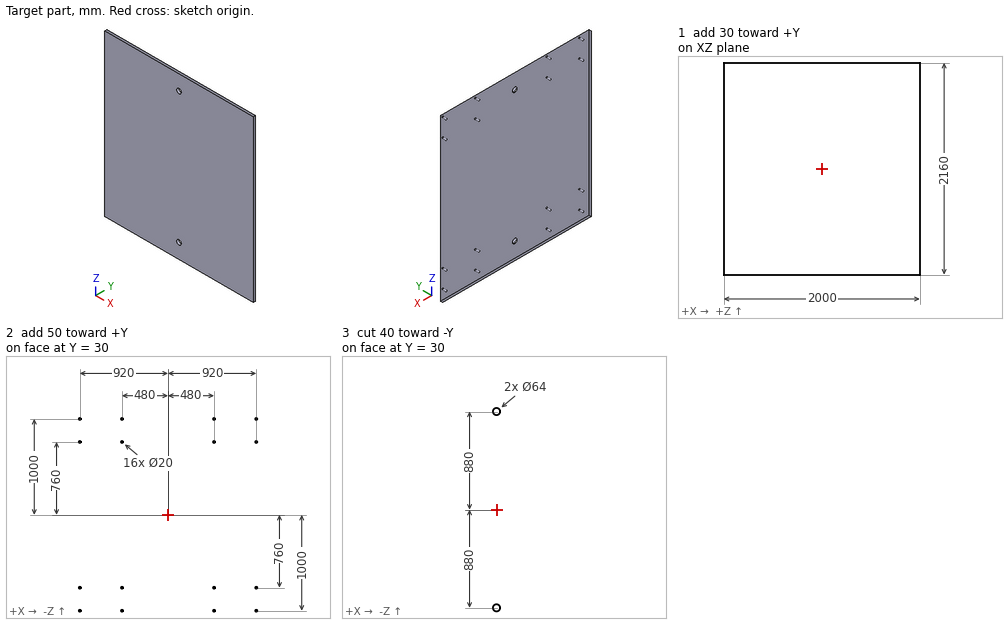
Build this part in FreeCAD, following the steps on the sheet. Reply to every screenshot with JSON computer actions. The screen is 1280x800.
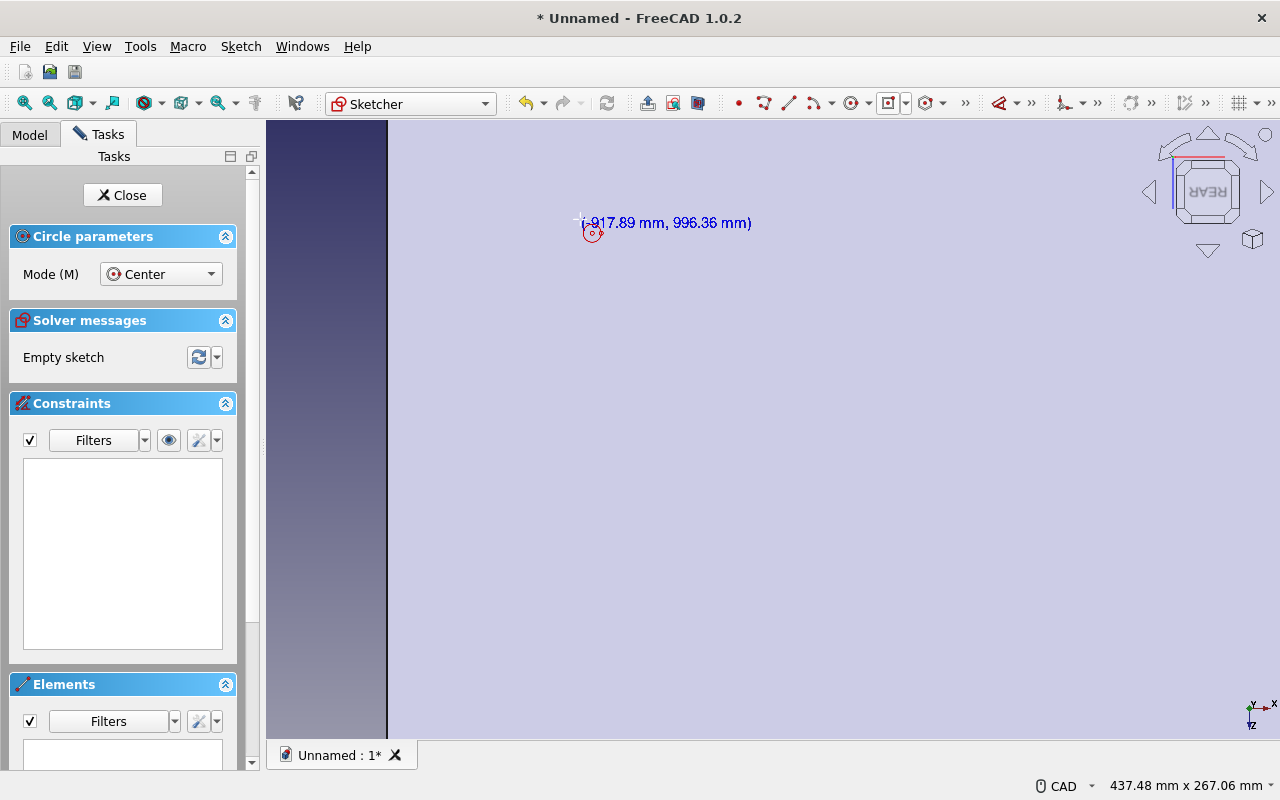
{"action": "scroll", "coordinate": [505, 219], "scroll_direction": "down", "scroll_amount": 12}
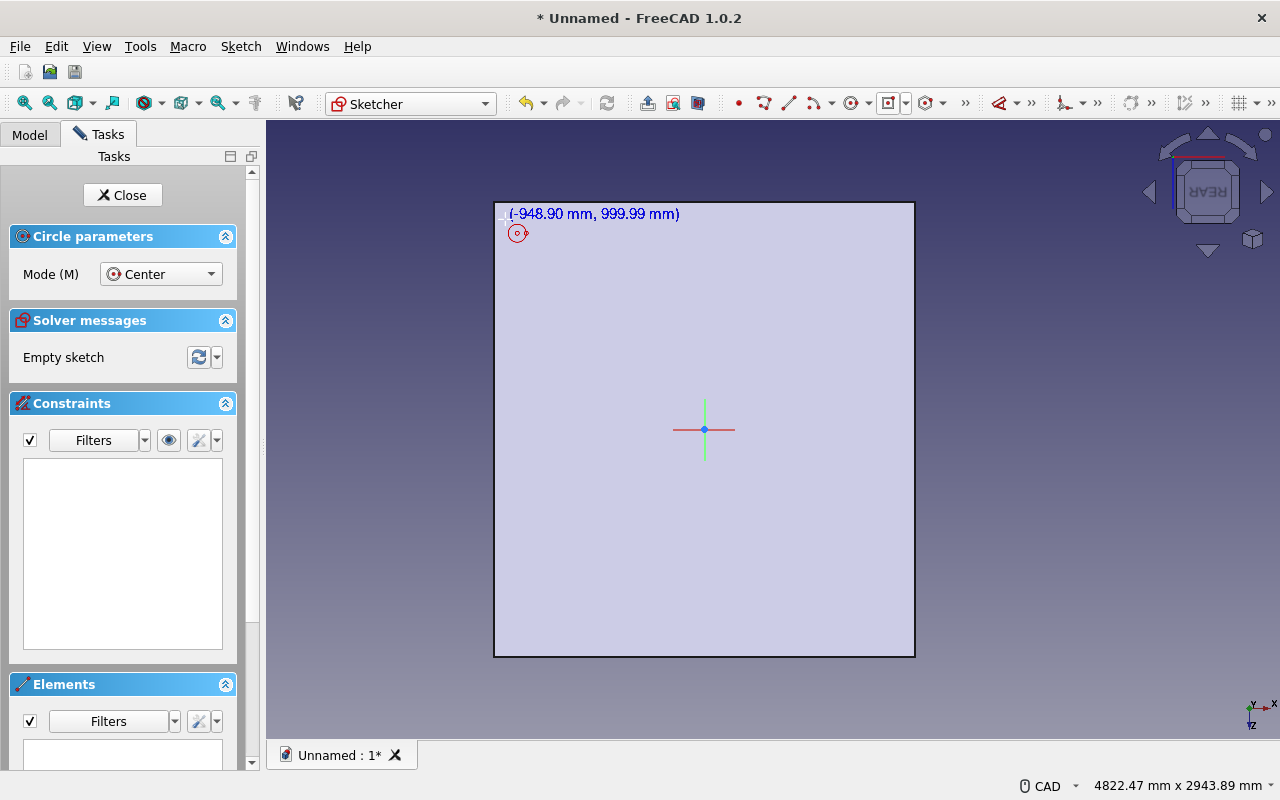
{"action": "left_click", "coordinate": [511, 219]}
{"action": "mouse_move", "coordinate": [513, 218]}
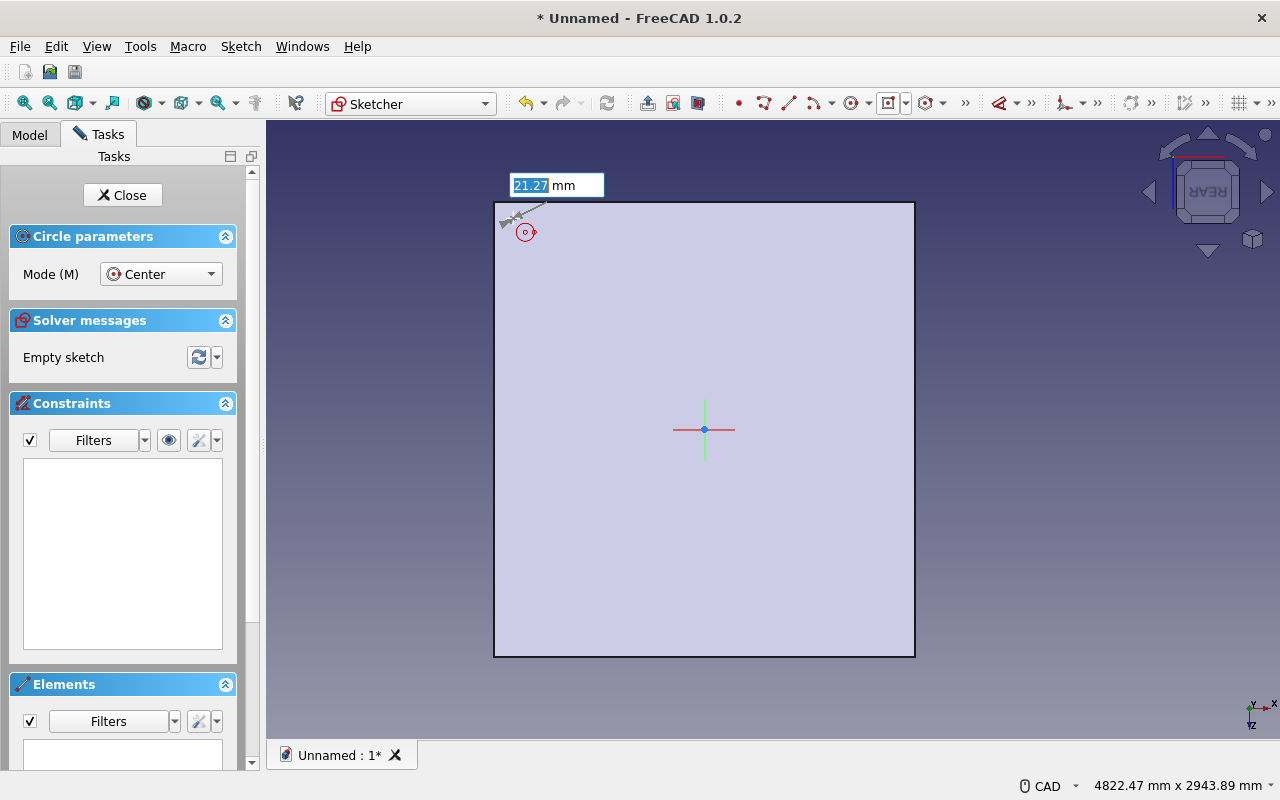
{"action": "type", "text": "20"}
{"action": "key", "text": "Return"}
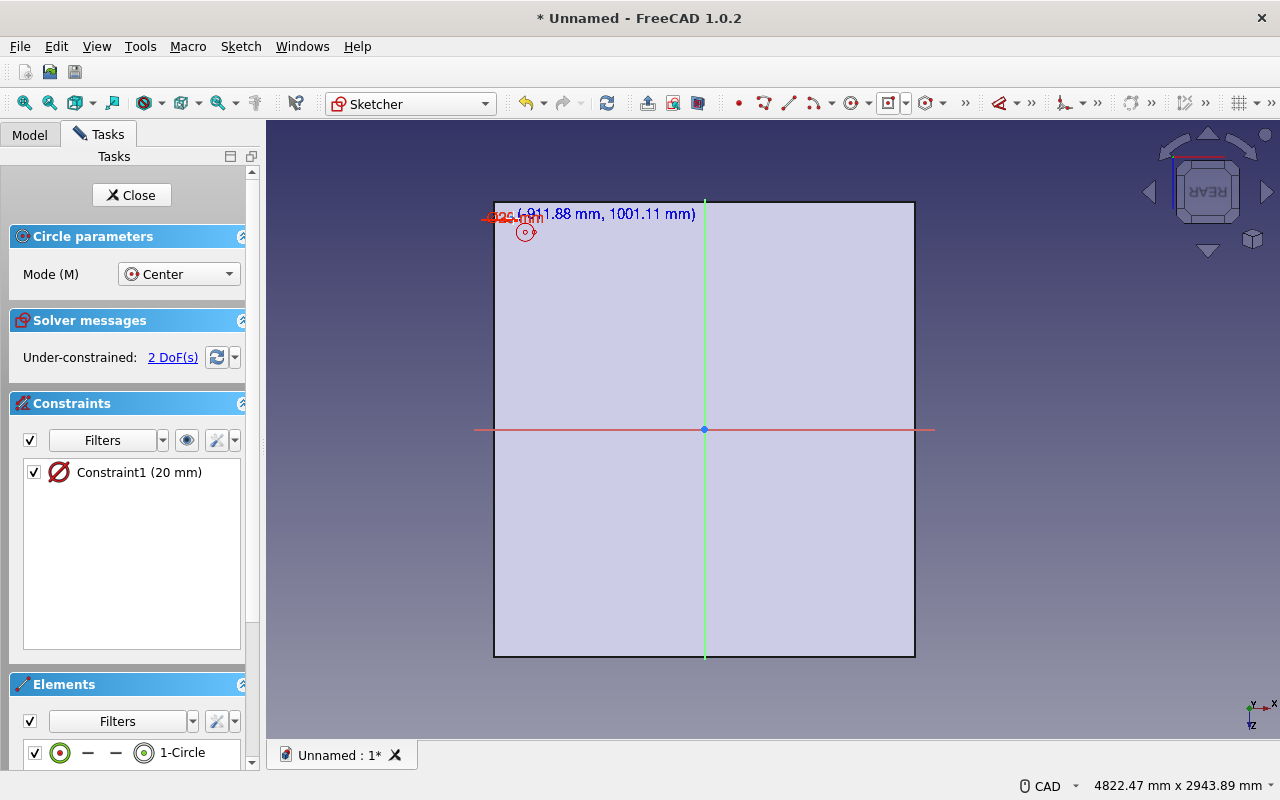
{"action": "scroll", "coordinate": [511, 270], "scroll_direction": "up", "scroll_amount": 12}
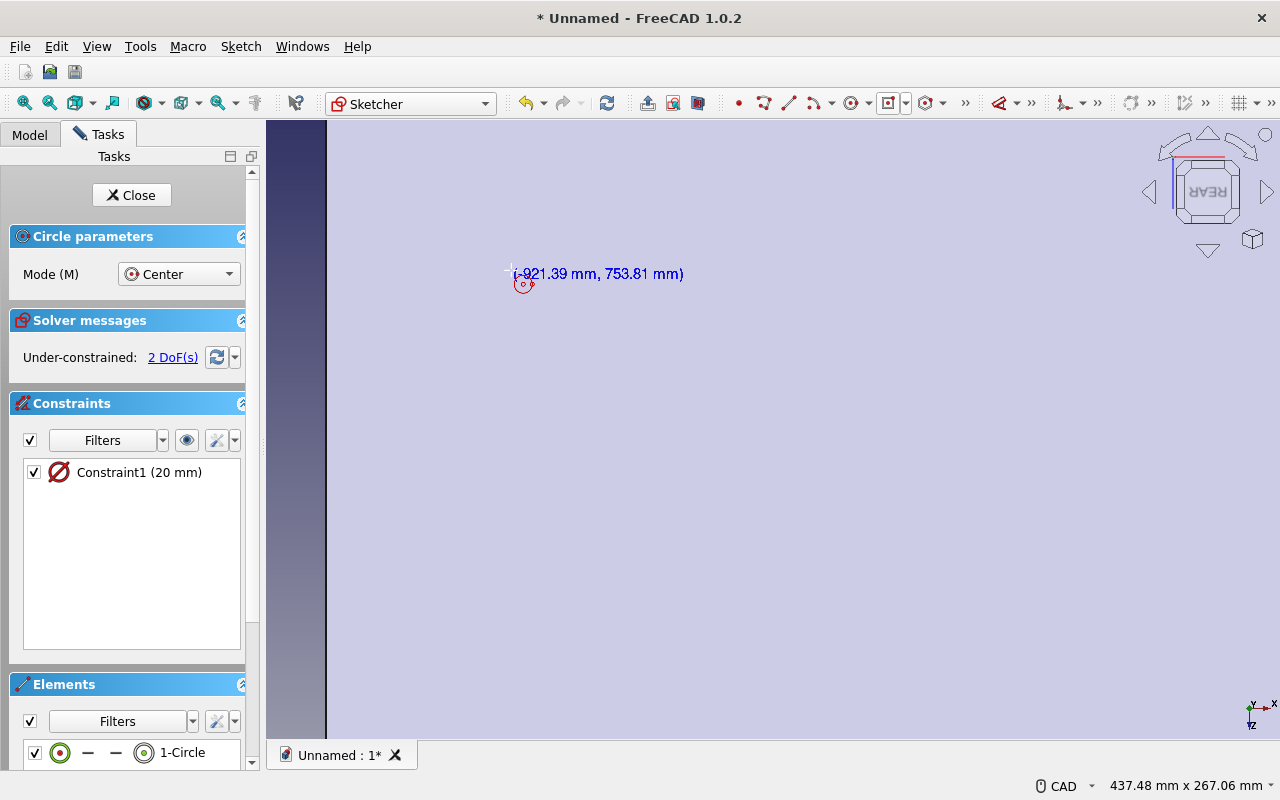
{"action": "scroll", "coordinate": [511, 270], "scroll_direction": "down", "scroll_amount": 12}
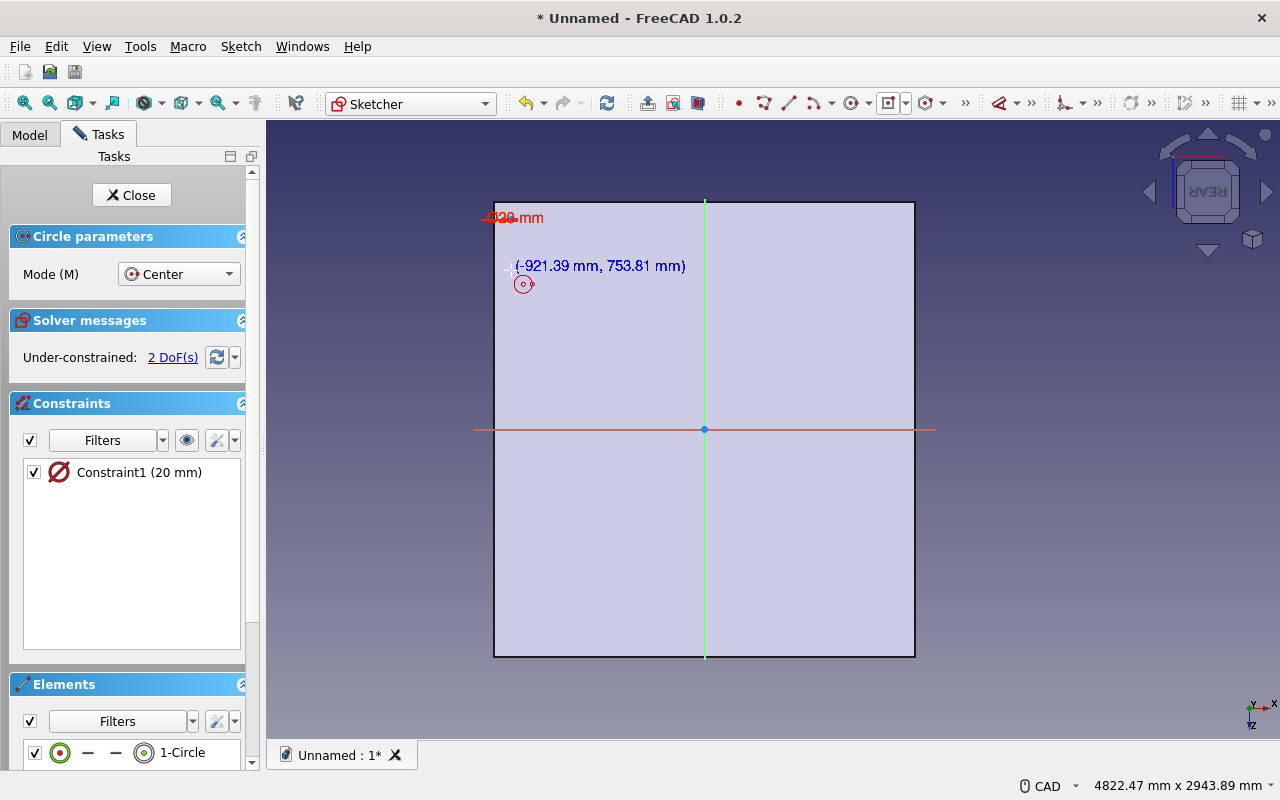
{"action": "left_click", "coordinate": [511, 270]}
{"action": "mouse_move", "coordinate": [513, 268]}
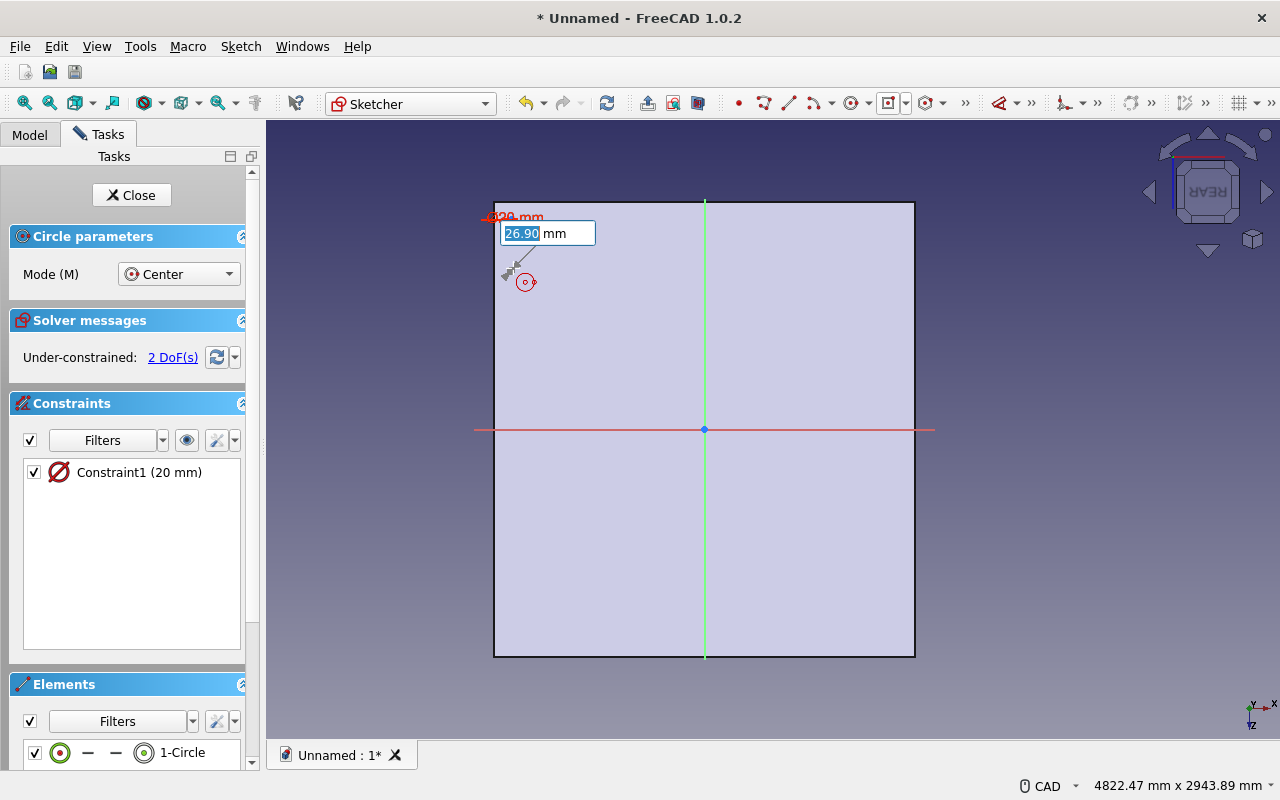
{"action": "type", "text": "20"}
{"action": "key", "text": "Return"}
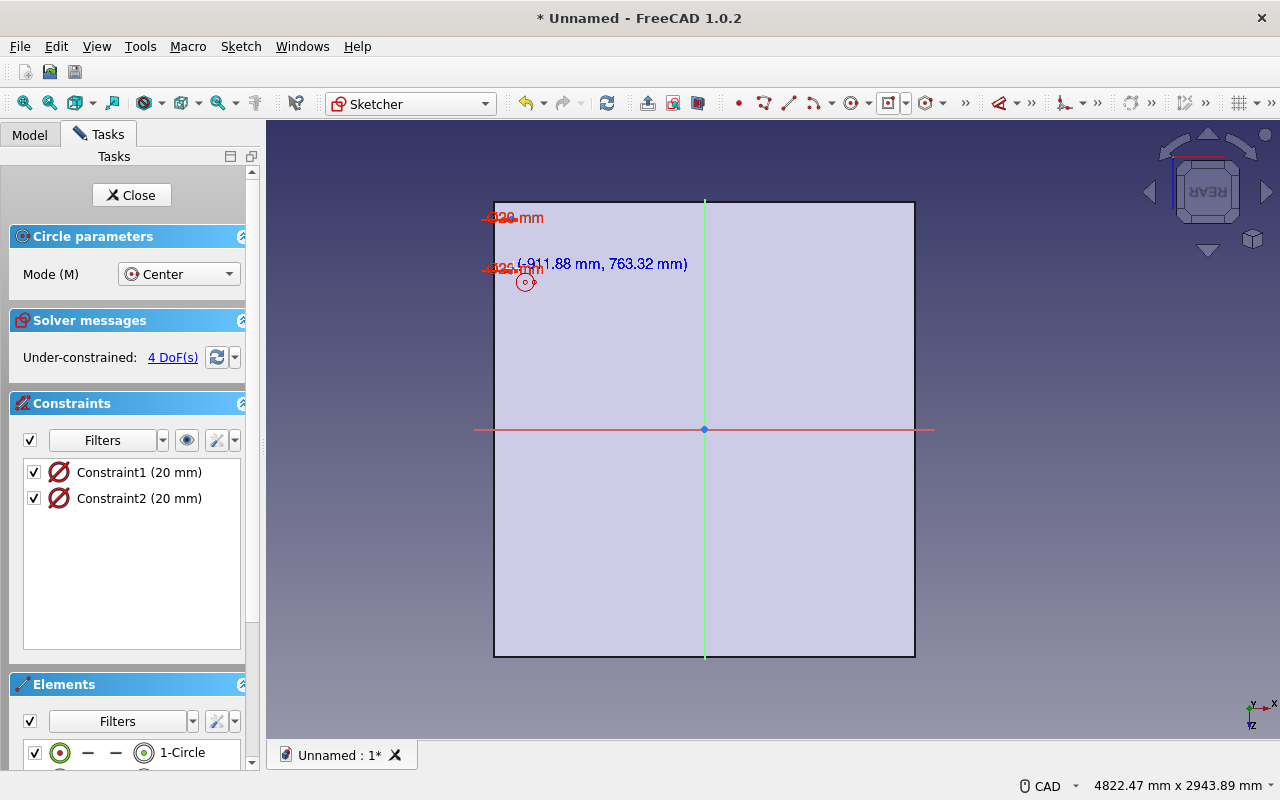
{"action": "scroll", "coordinate": [604, 219], "scroll_direction": "up", "scroll_amount": 12}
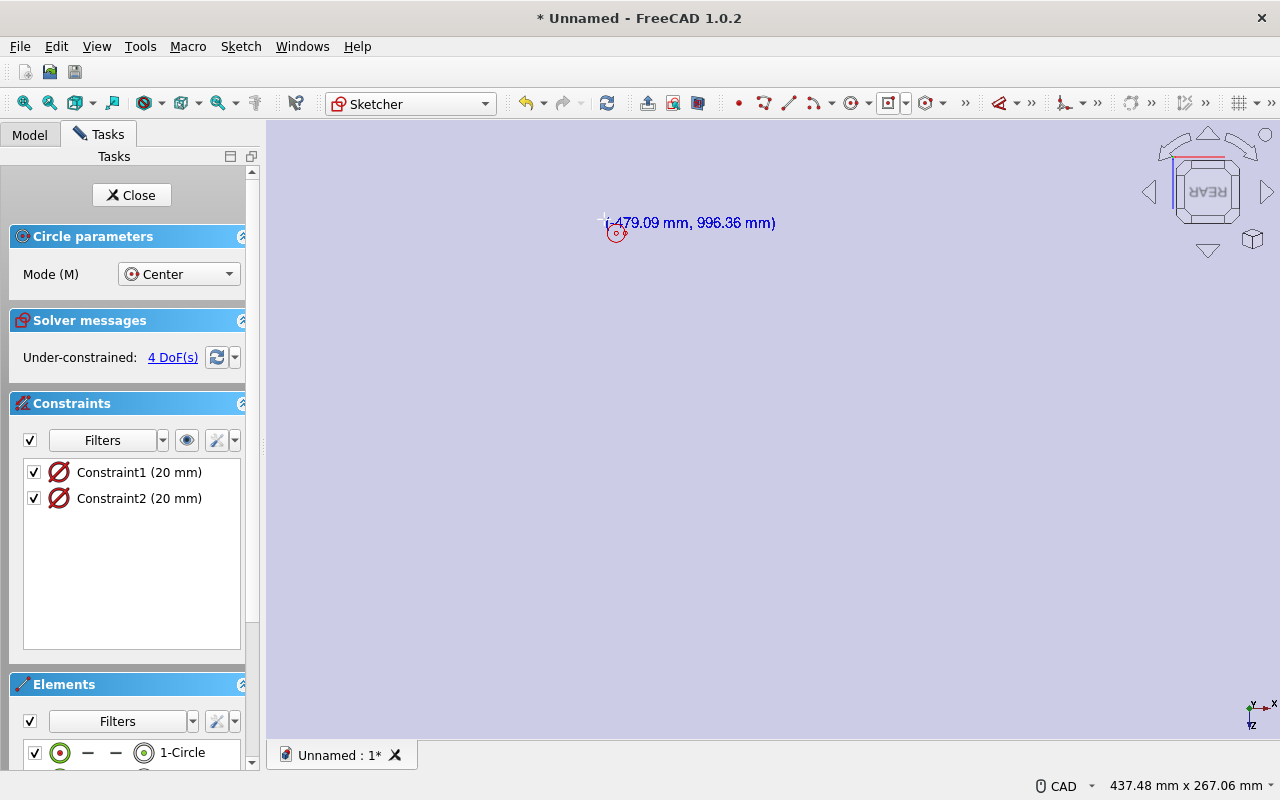
{"action": "scroll", "coordinate": [604, 219], "scroll_direction": "down", "scroll_amount": 12}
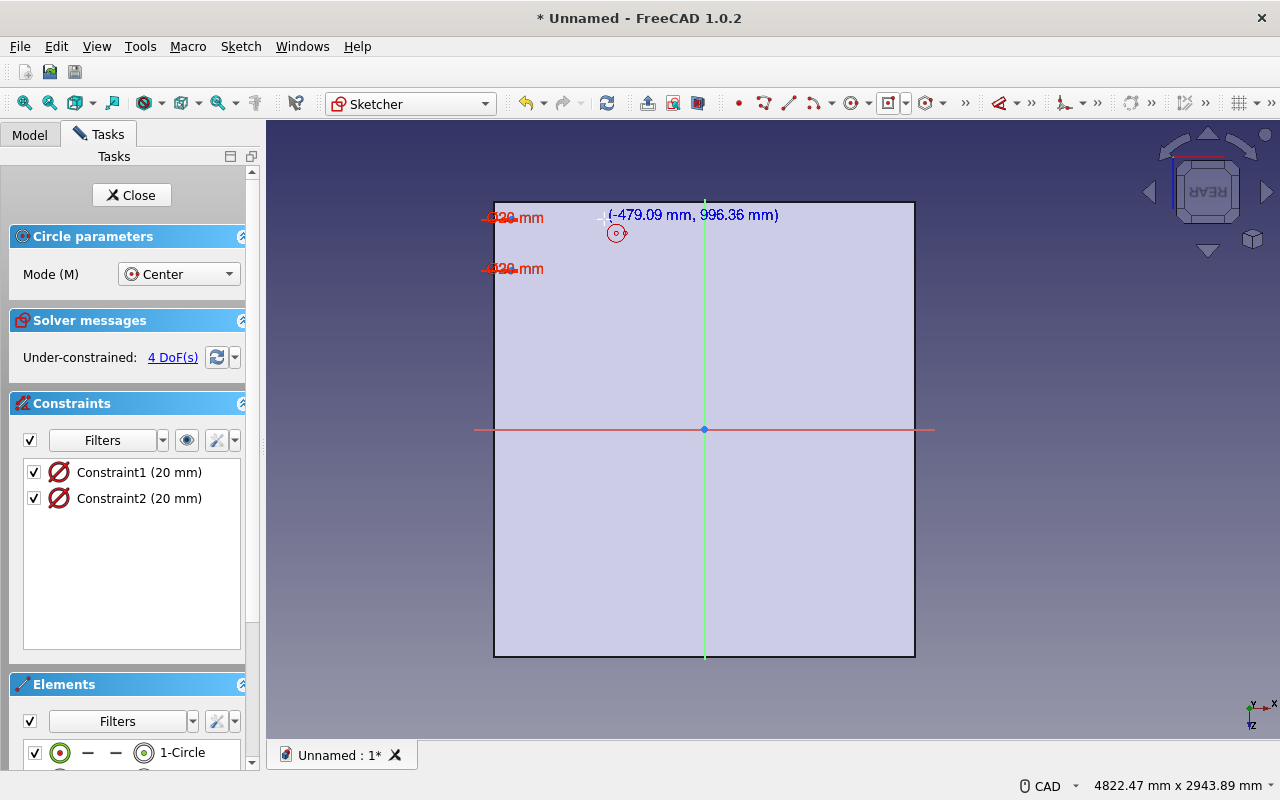
{"action": "left_click", "coordinate": [604, 219]}
{"action": "mouse_move", "coordinate": [605, 218]}